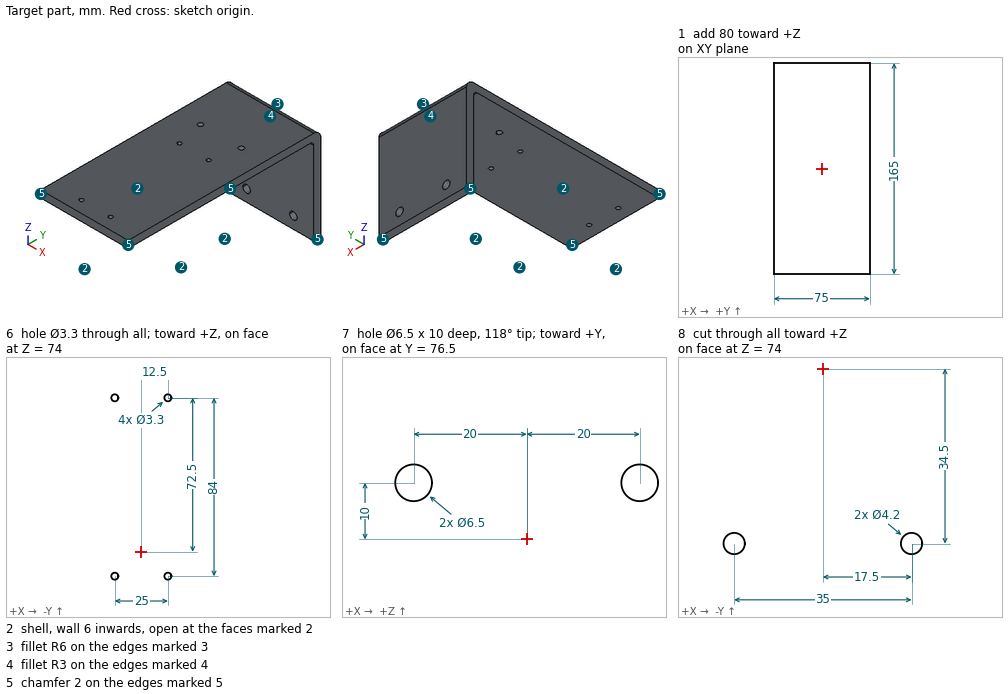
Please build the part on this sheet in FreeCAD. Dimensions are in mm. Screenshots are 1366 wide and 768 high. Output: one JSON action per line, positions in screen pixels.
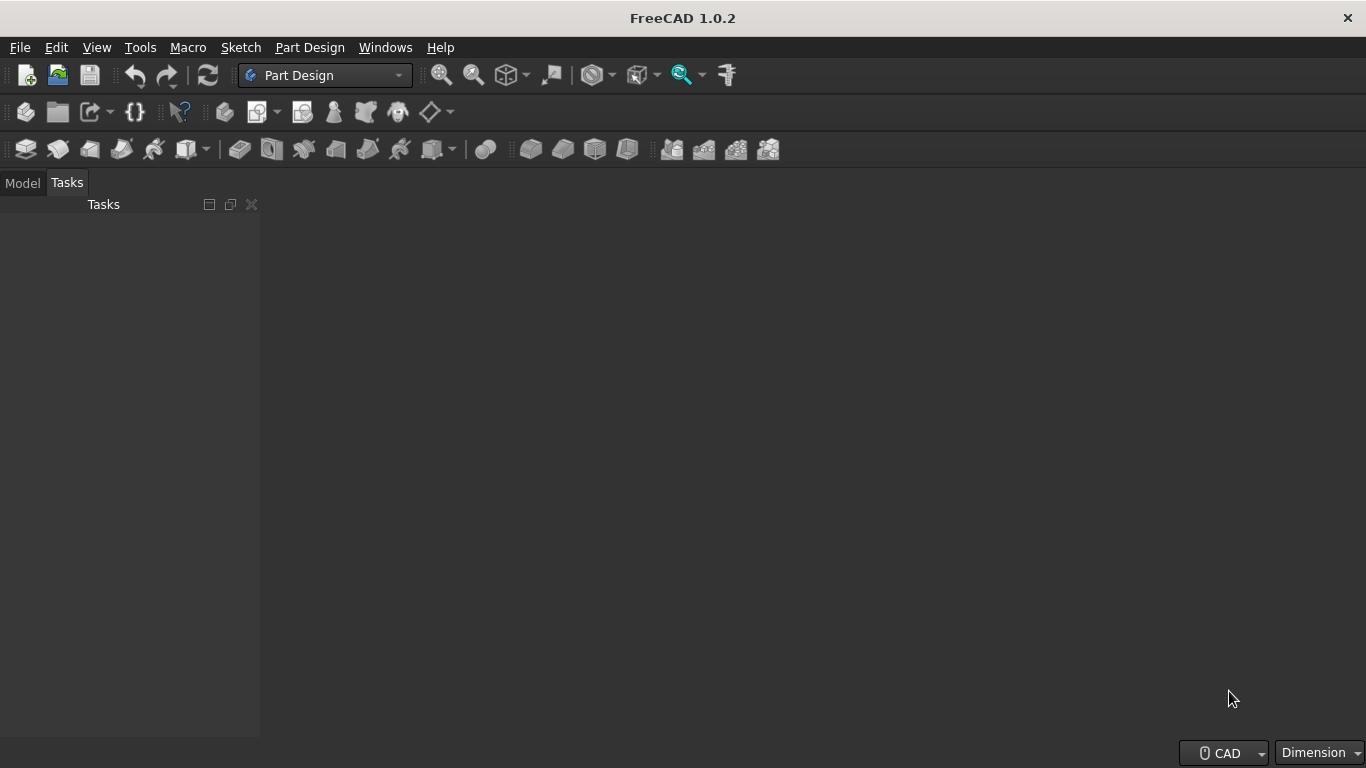
{"action": "left_click", "coordinate": [26, 76]}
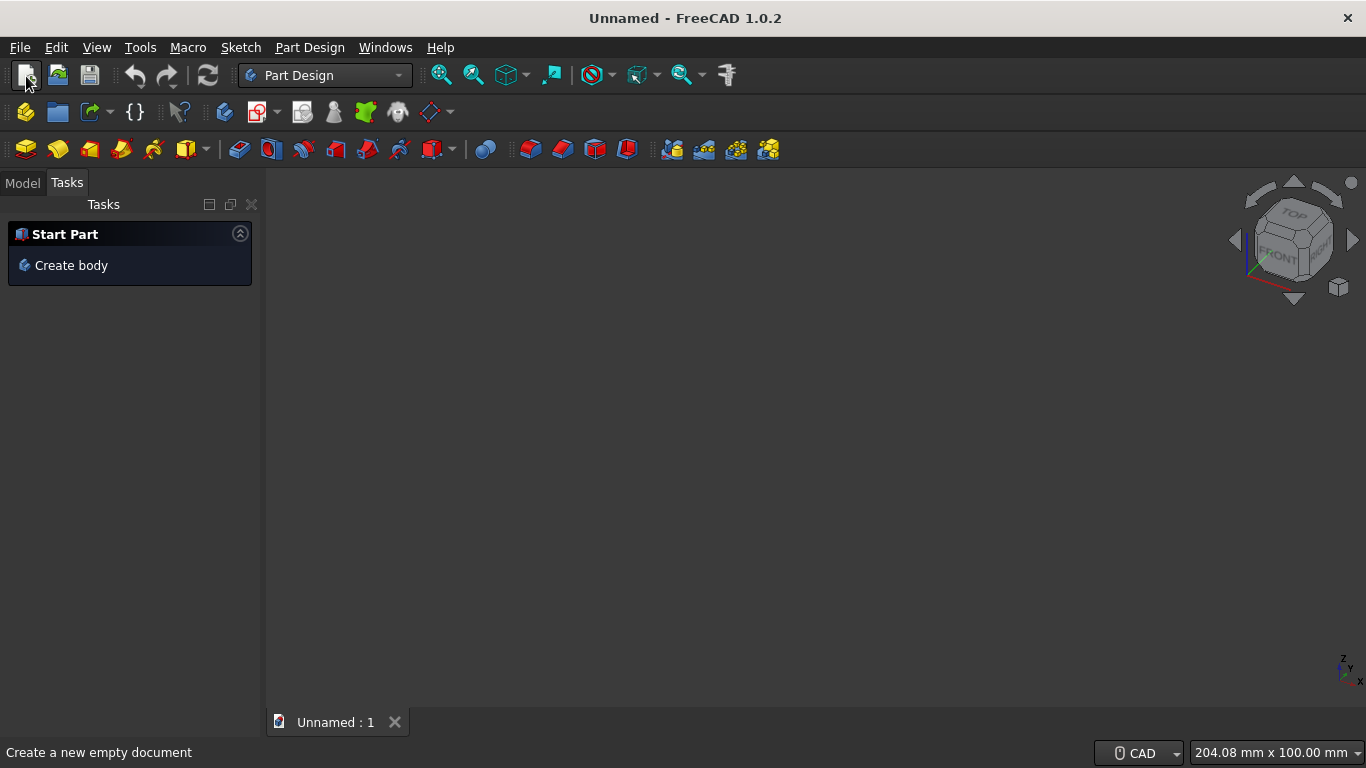
{"action": "left_click", "coordinate": [258, 112]}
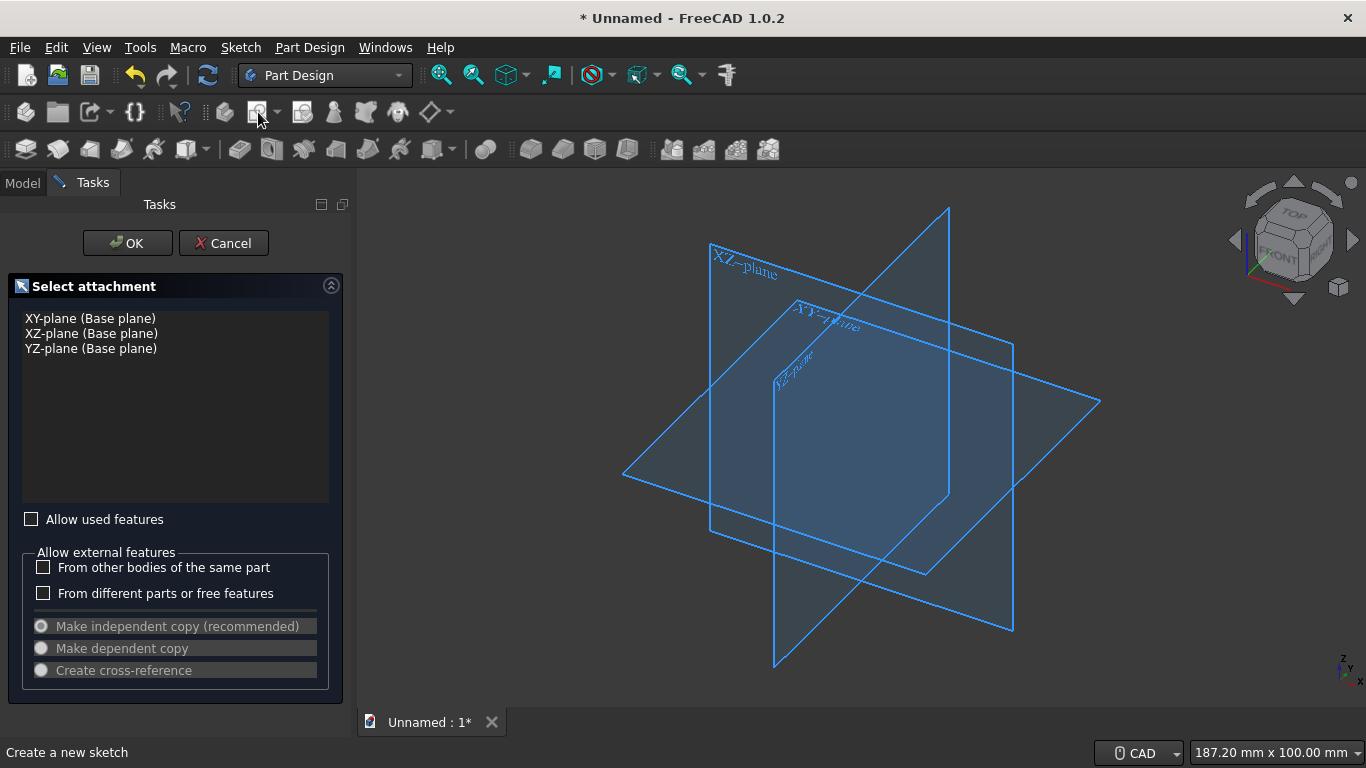
{"action": "left_click", "coordinate": [82, 318]}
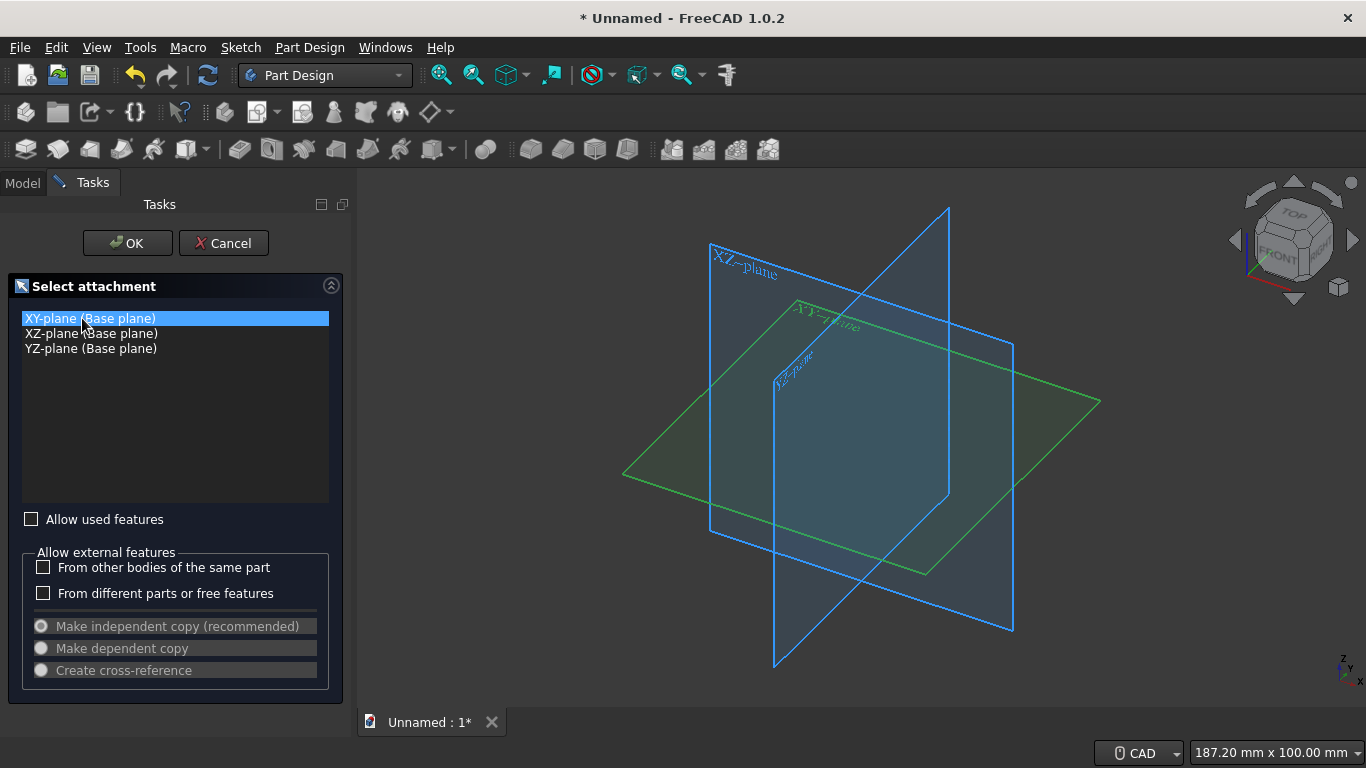
{"action": "left_click", "coordinate": [128, 243]}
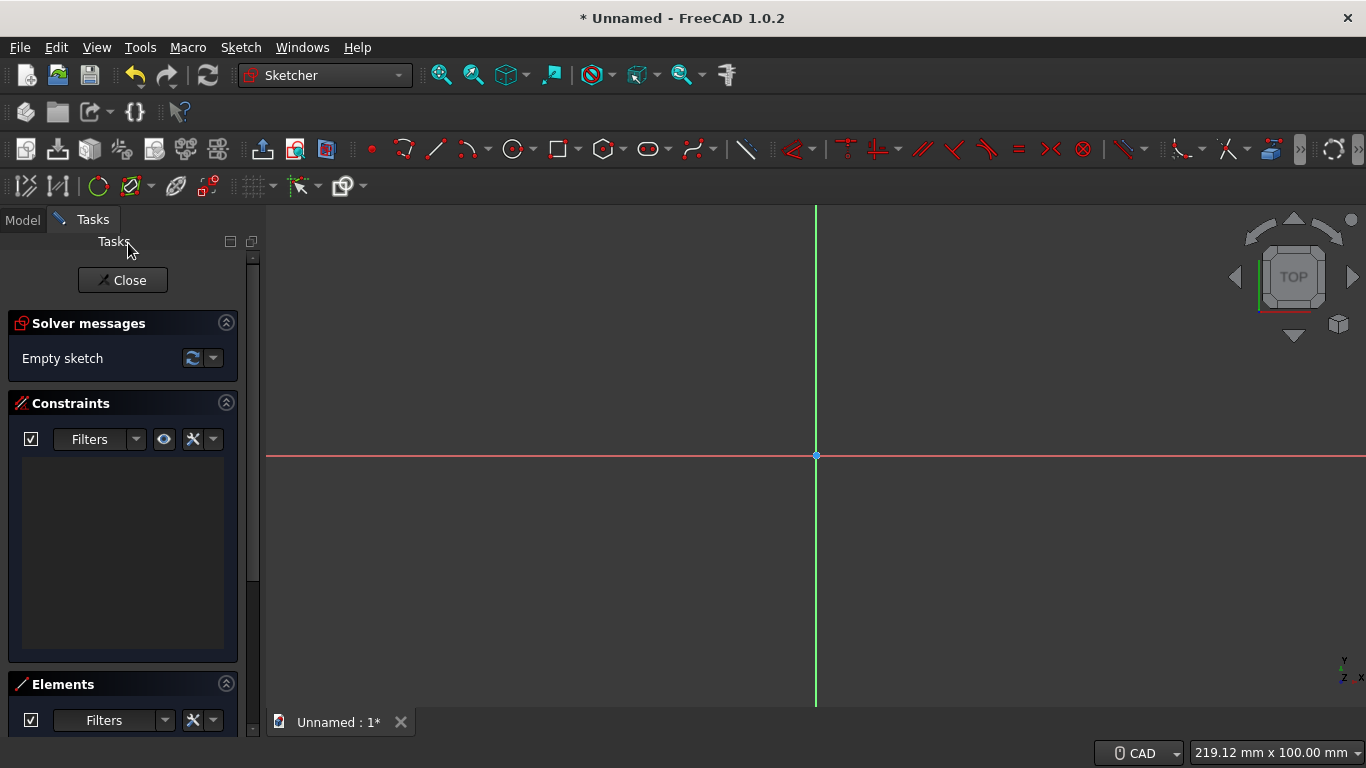
{"action": "scroll", "coordinate": [708, 456], "scroll_direction": "down", "scroll_amount": 5}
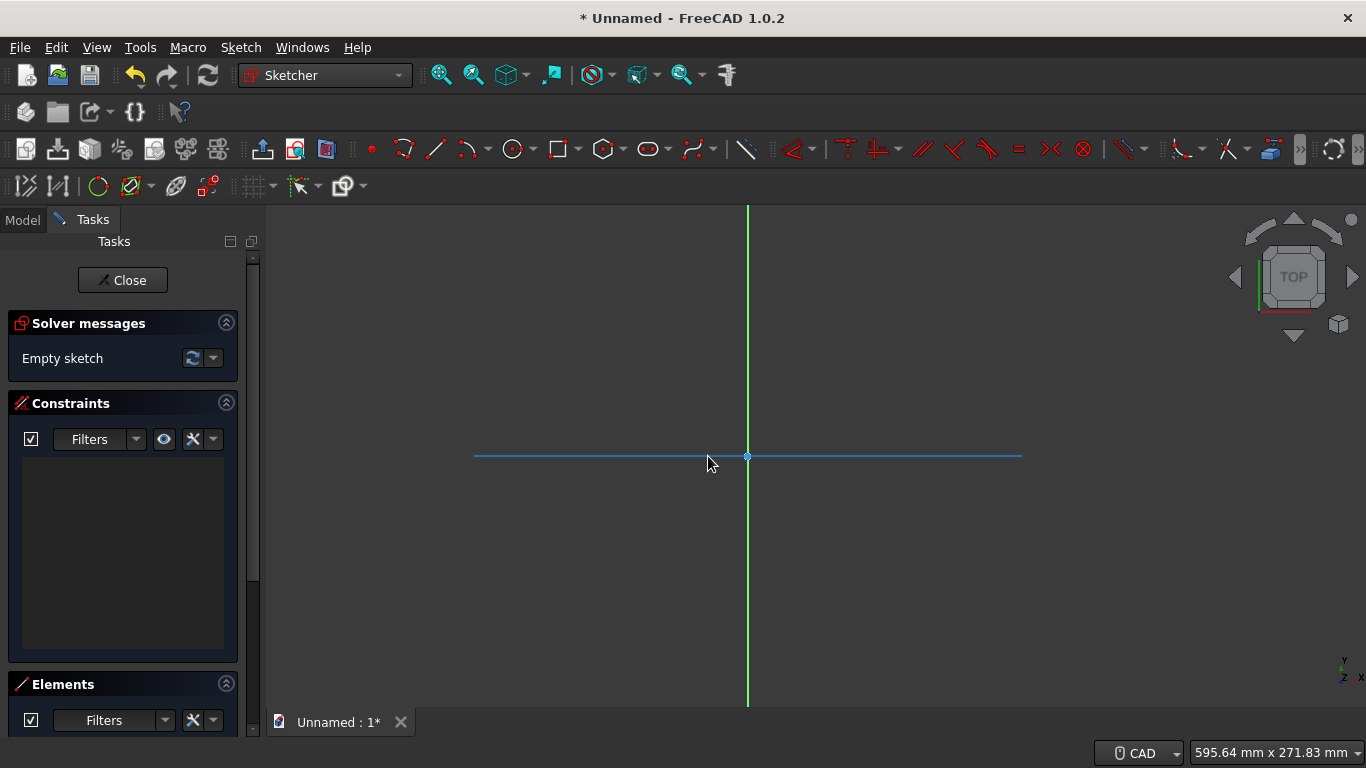
{"action": "key", "text": "g v"}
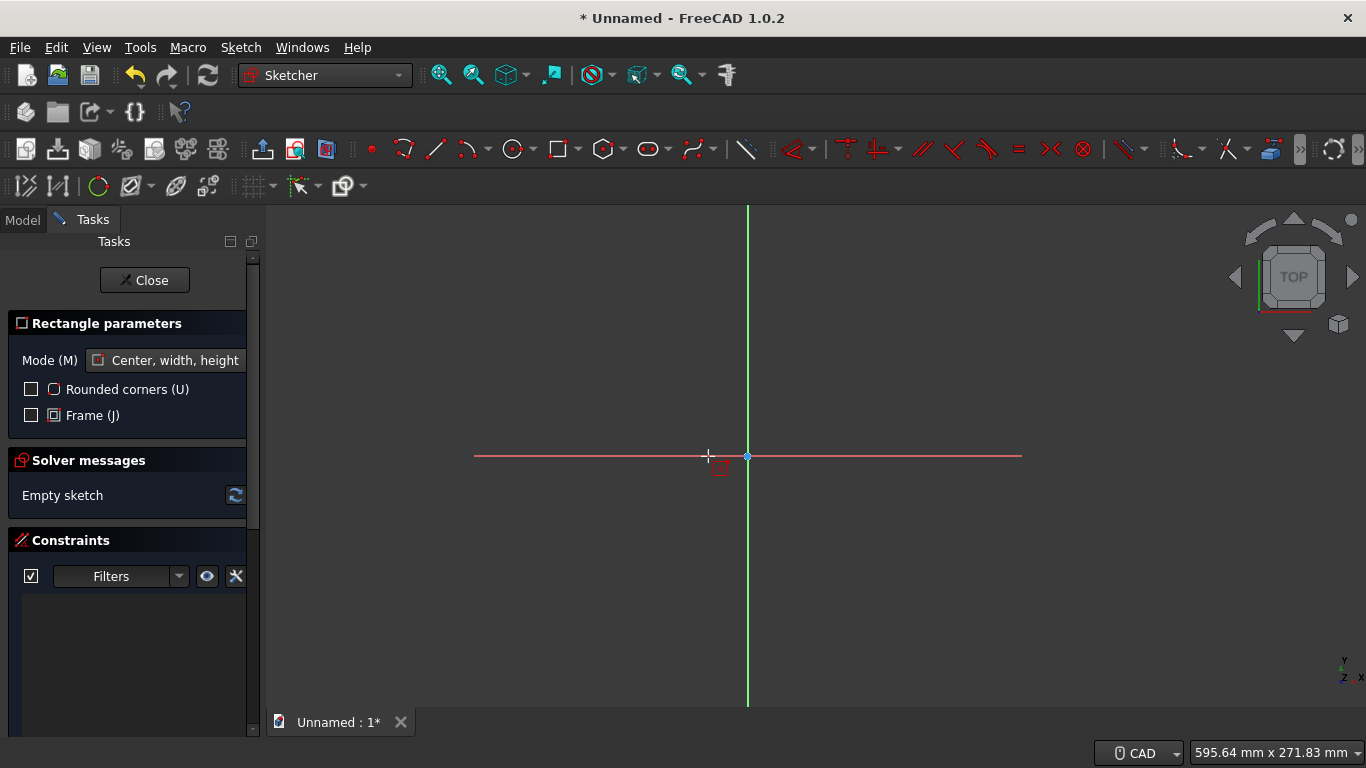
{"action": "left_click", "coordinate": [748, 456]}
{"action": "left_click", "coordinate": [817, 304]}
{"action": "key", "text": "Escape"}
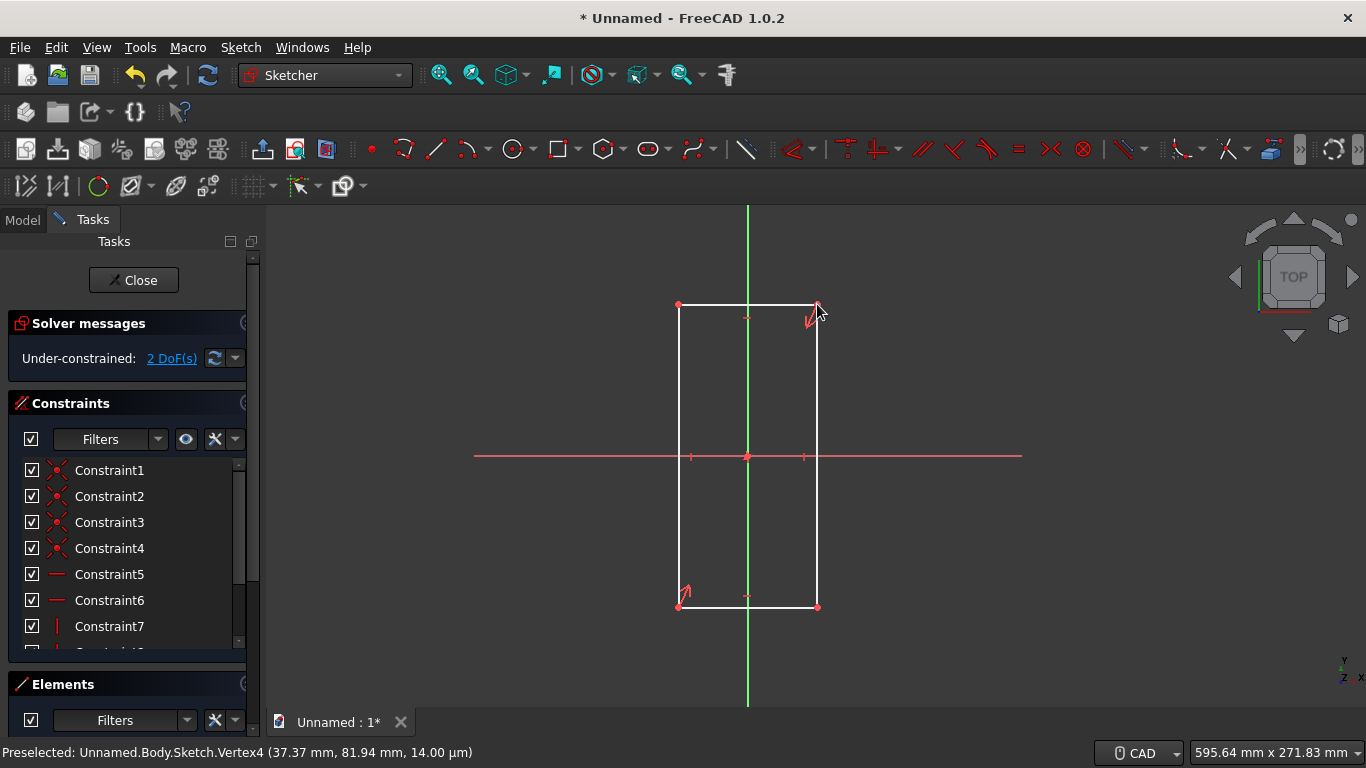
{"action": "left_click", "coordinate": [792, 150]}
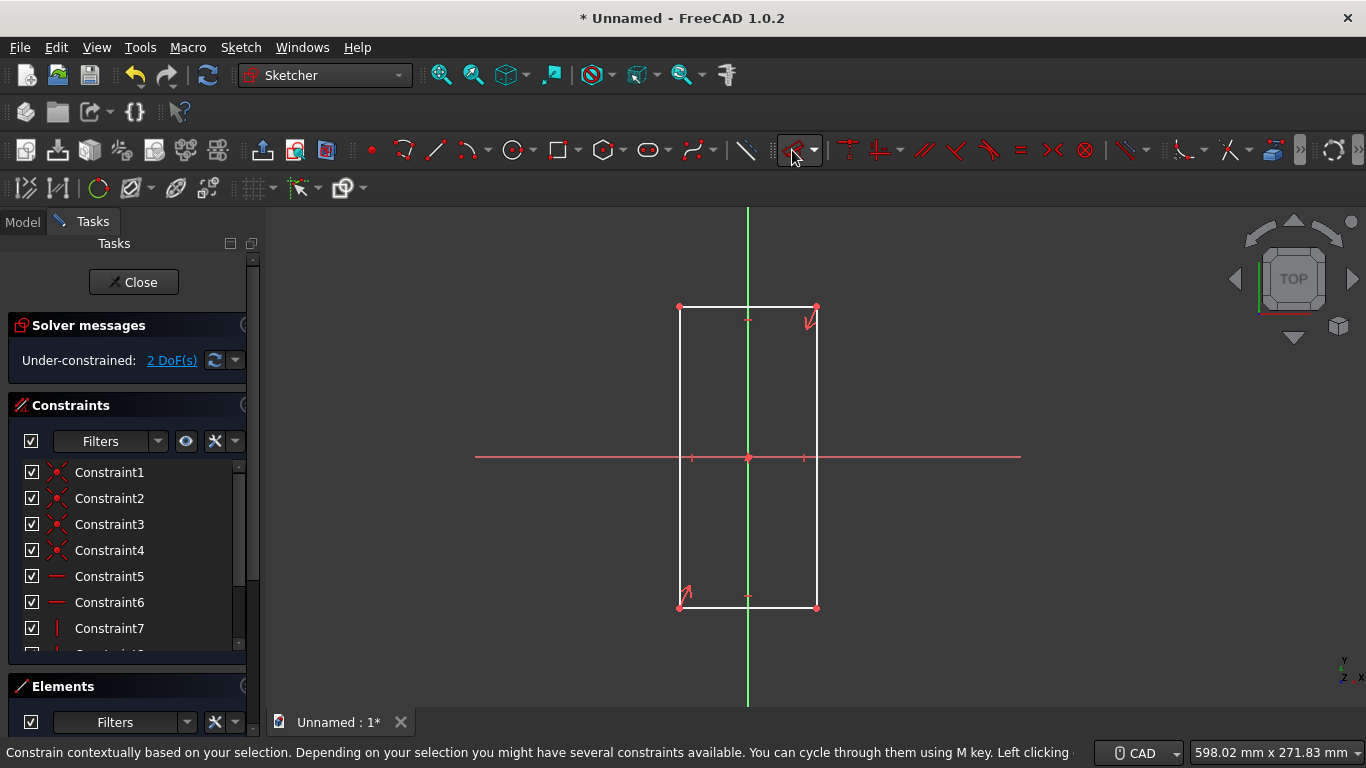
{"action": "left_click", "coordinate": [721, 608]}
{"action": "left_click", "coordinate": [717, 642]}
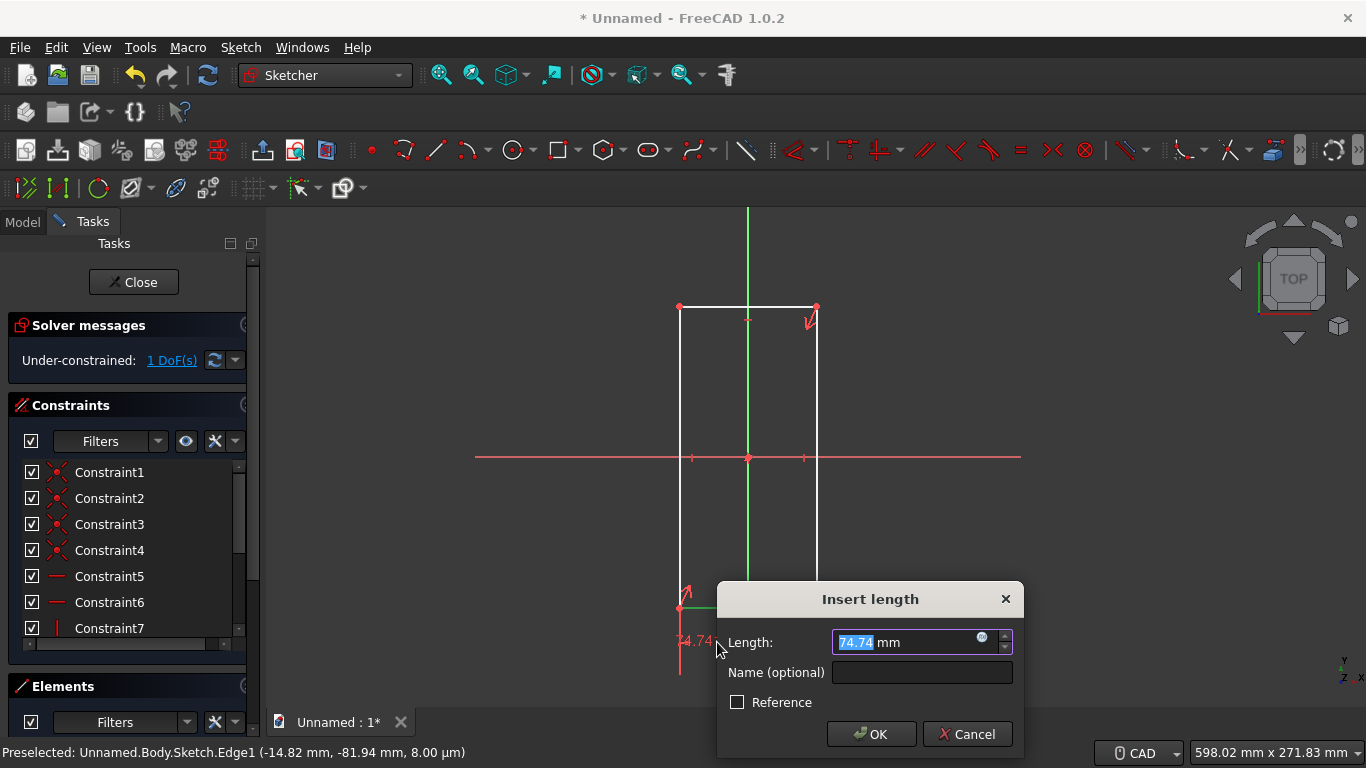
{"action": "type", "text": "75"}
{"action": "key", "text": "Return"}